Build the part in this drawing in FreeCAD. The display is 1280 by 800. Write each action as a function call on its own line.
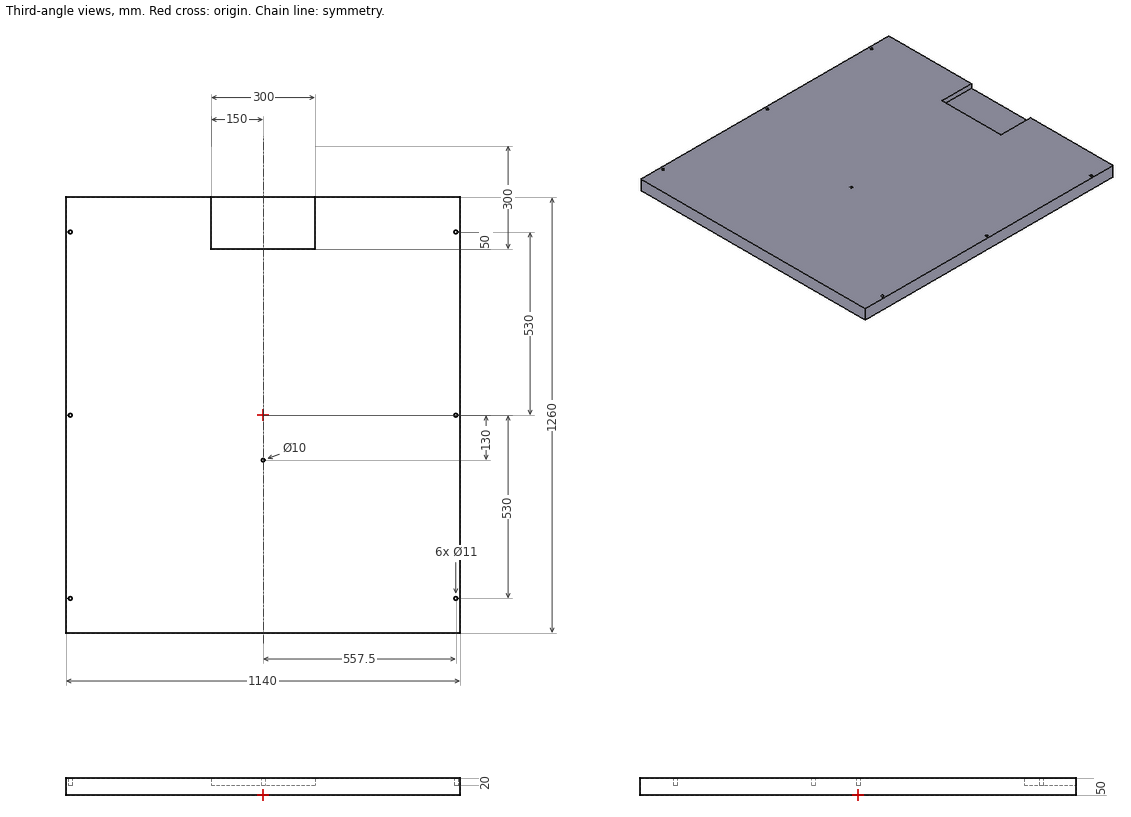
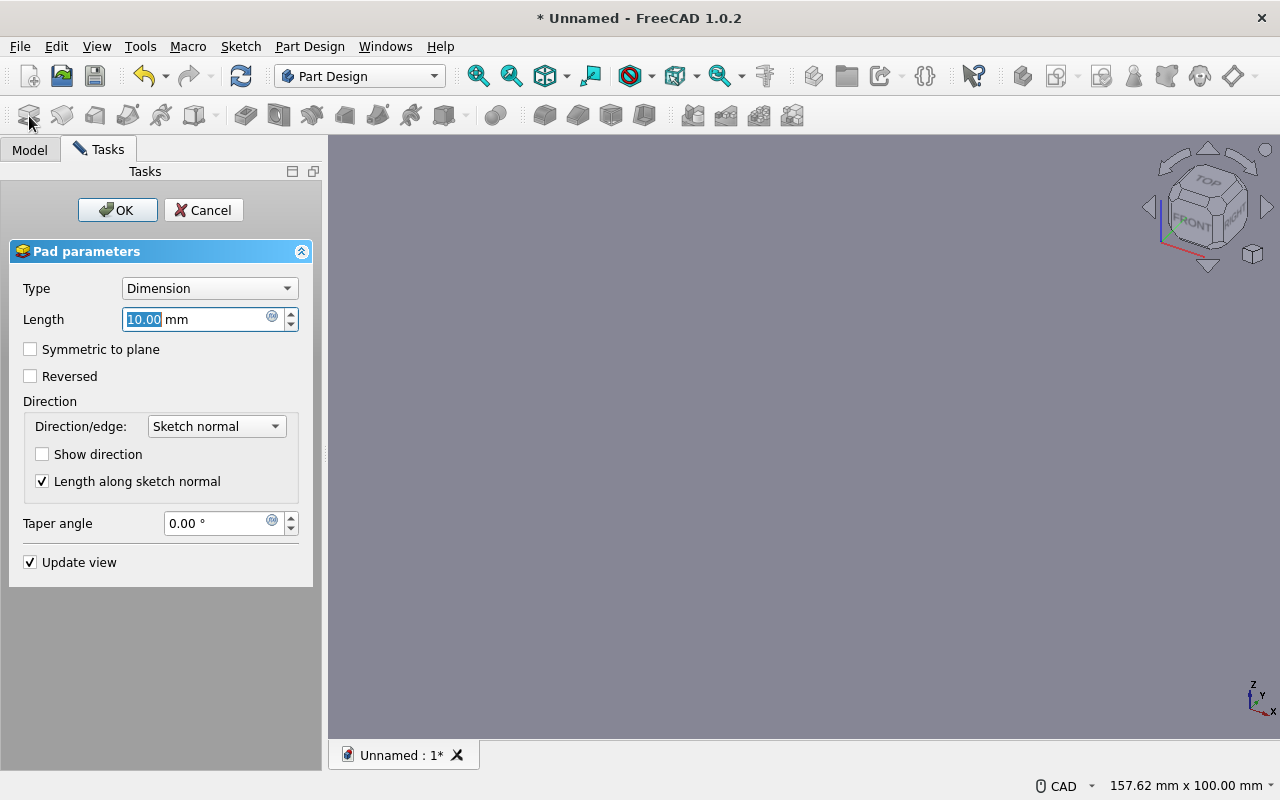
text(50)
key(Tab)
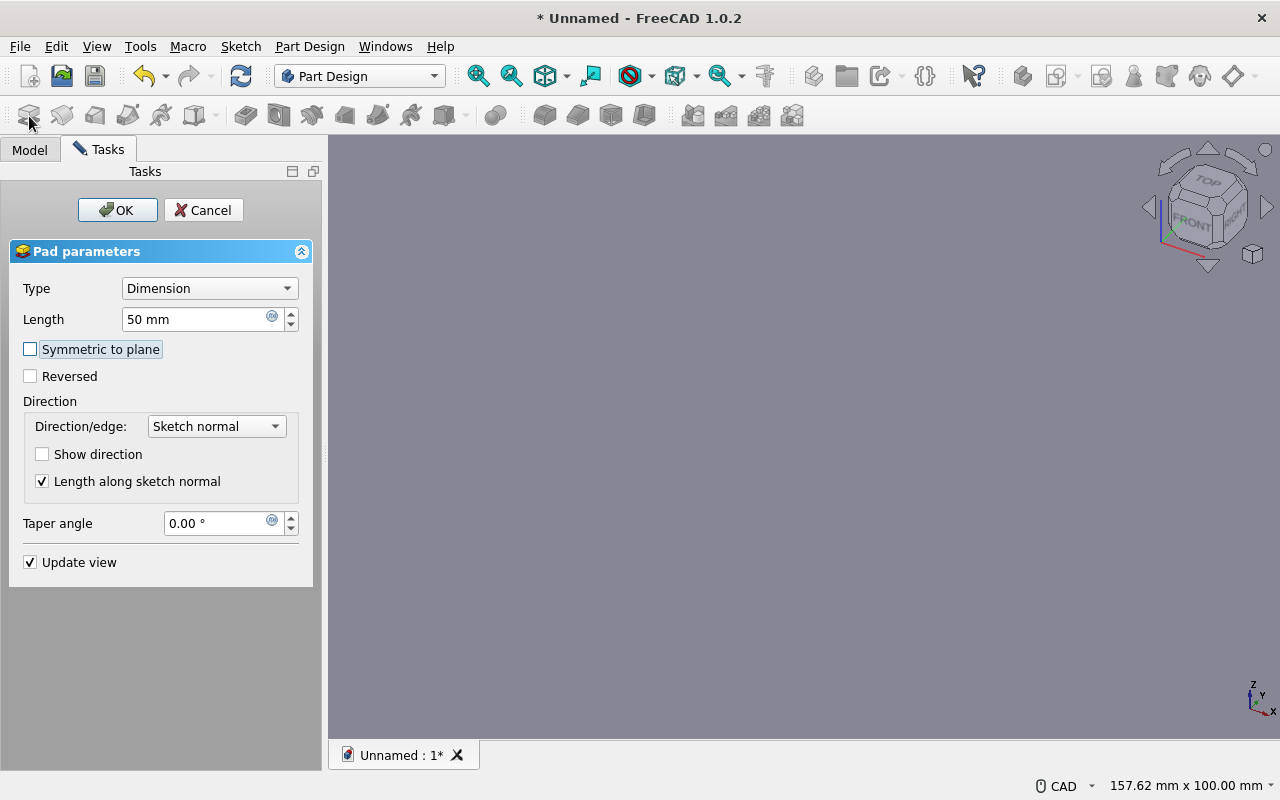
click(118, 210)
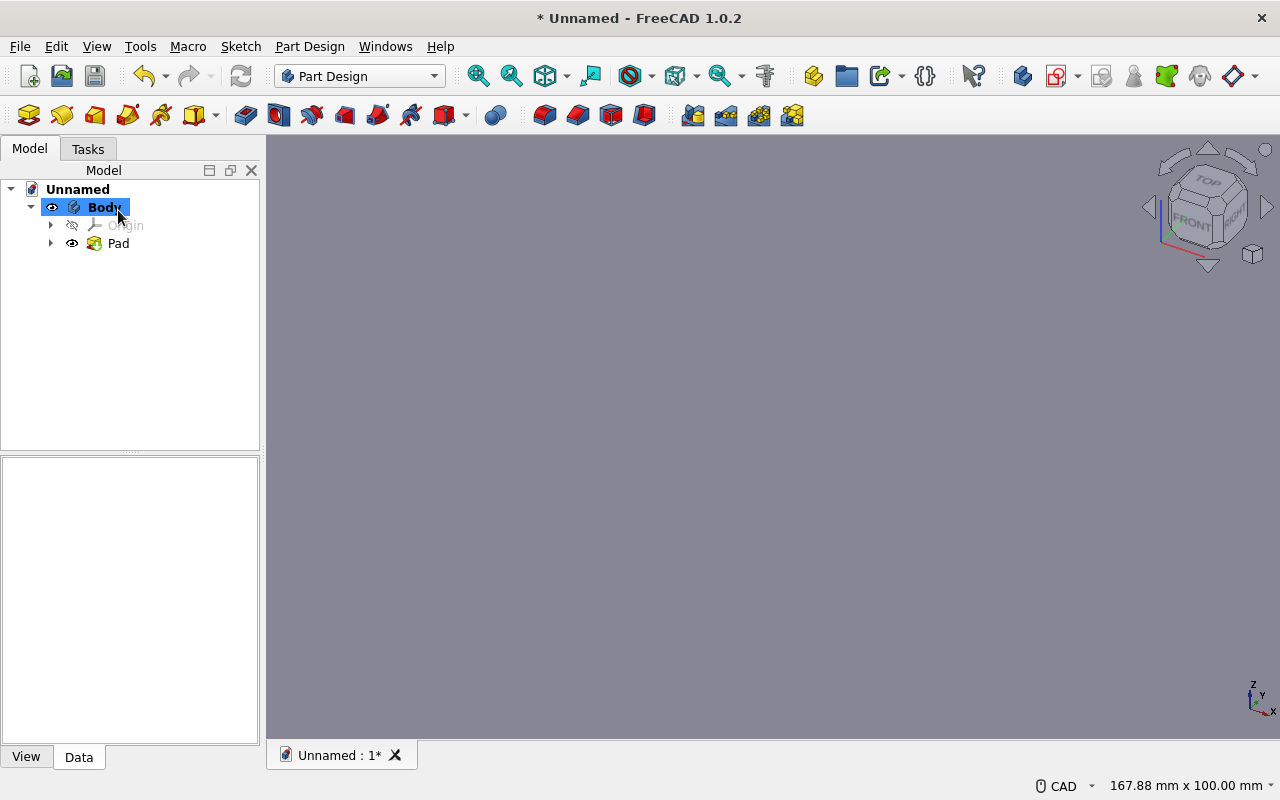
click(479, 76)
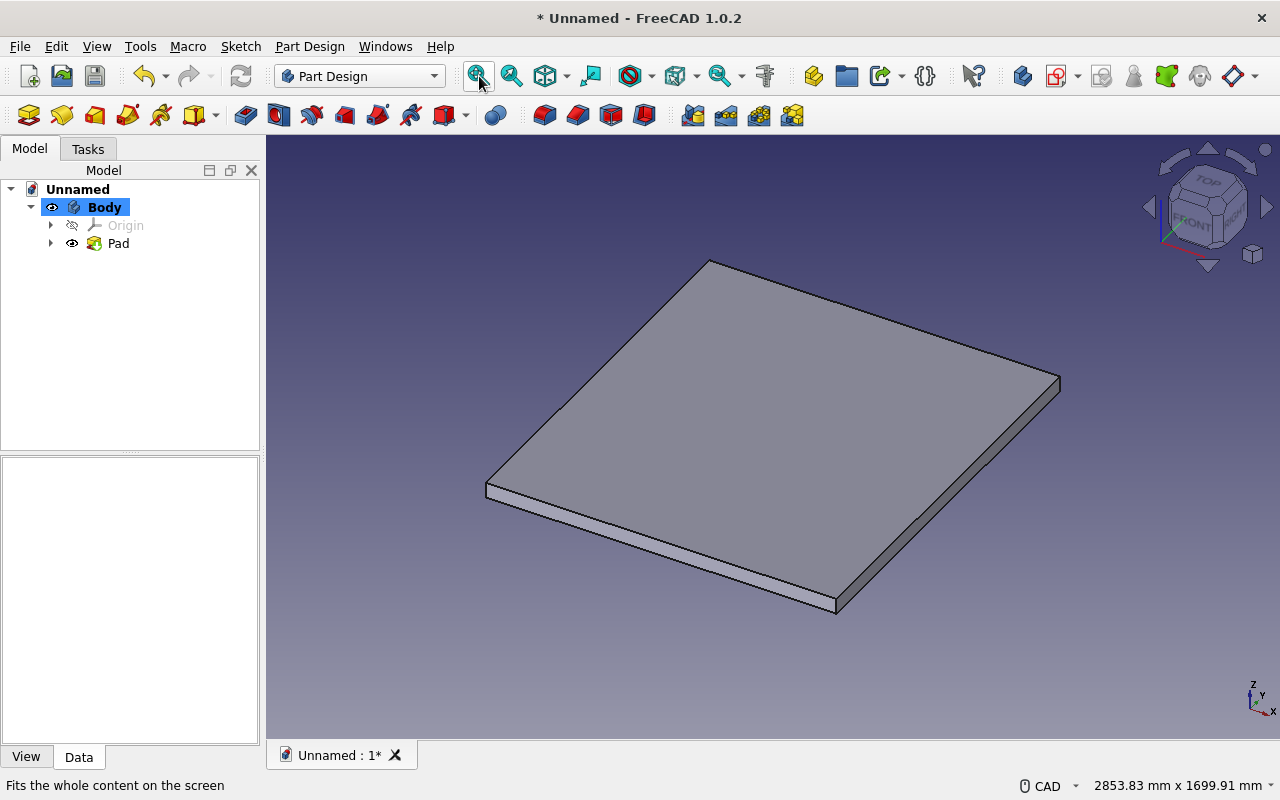
click(773, 429)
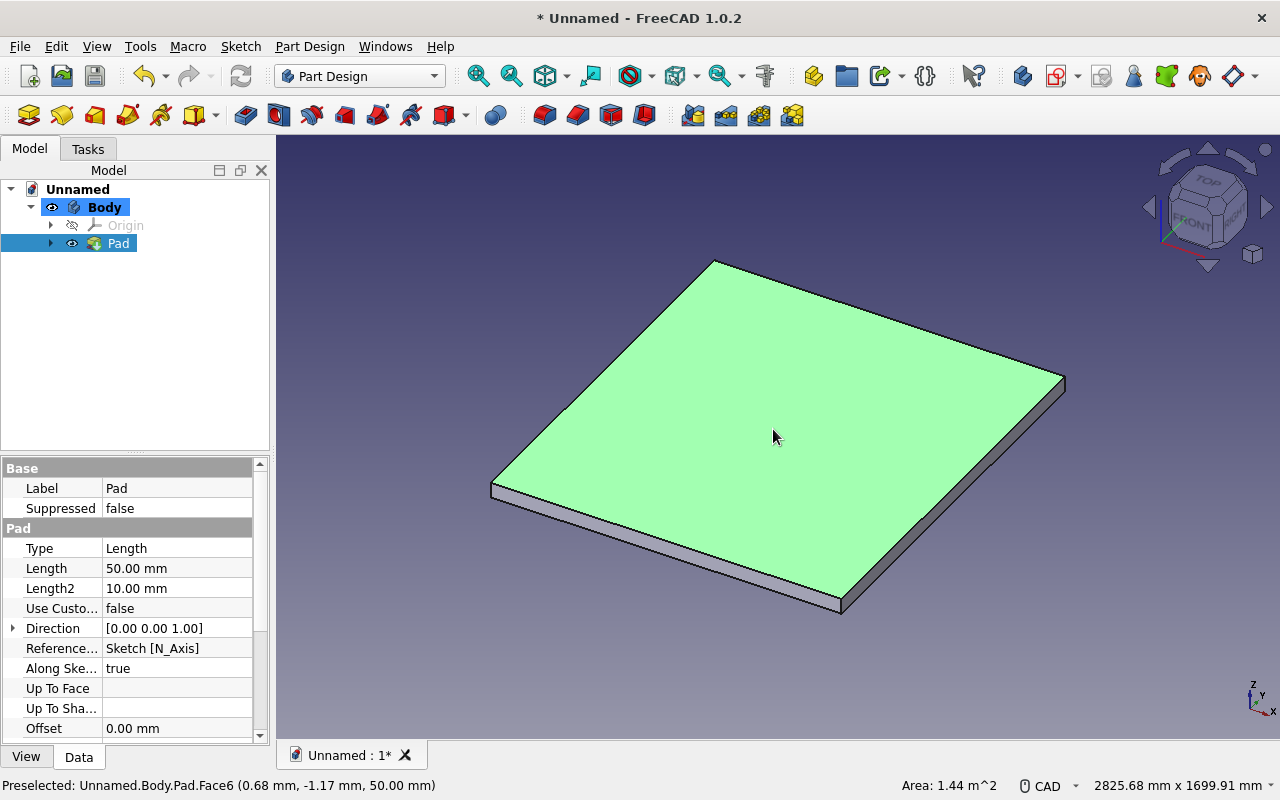
click(1056, 76)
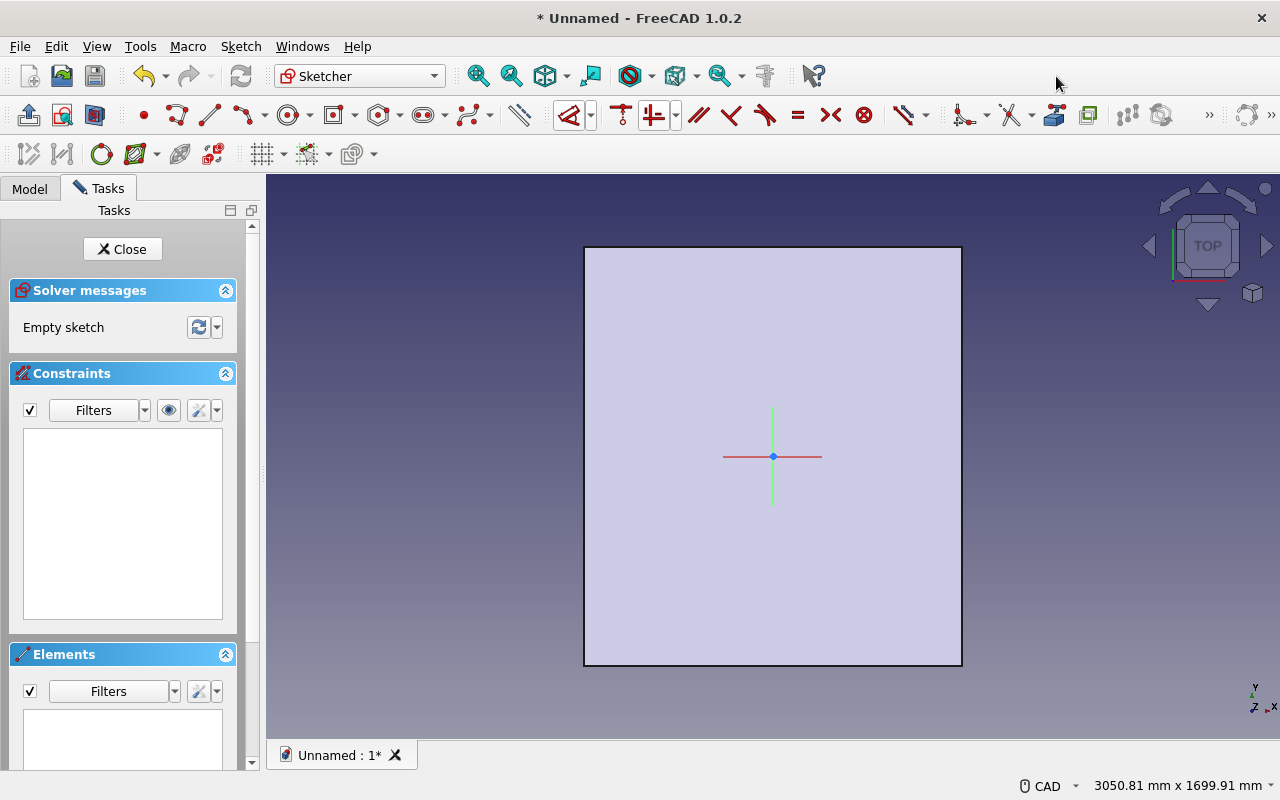
scroll(395, 640, down, 1)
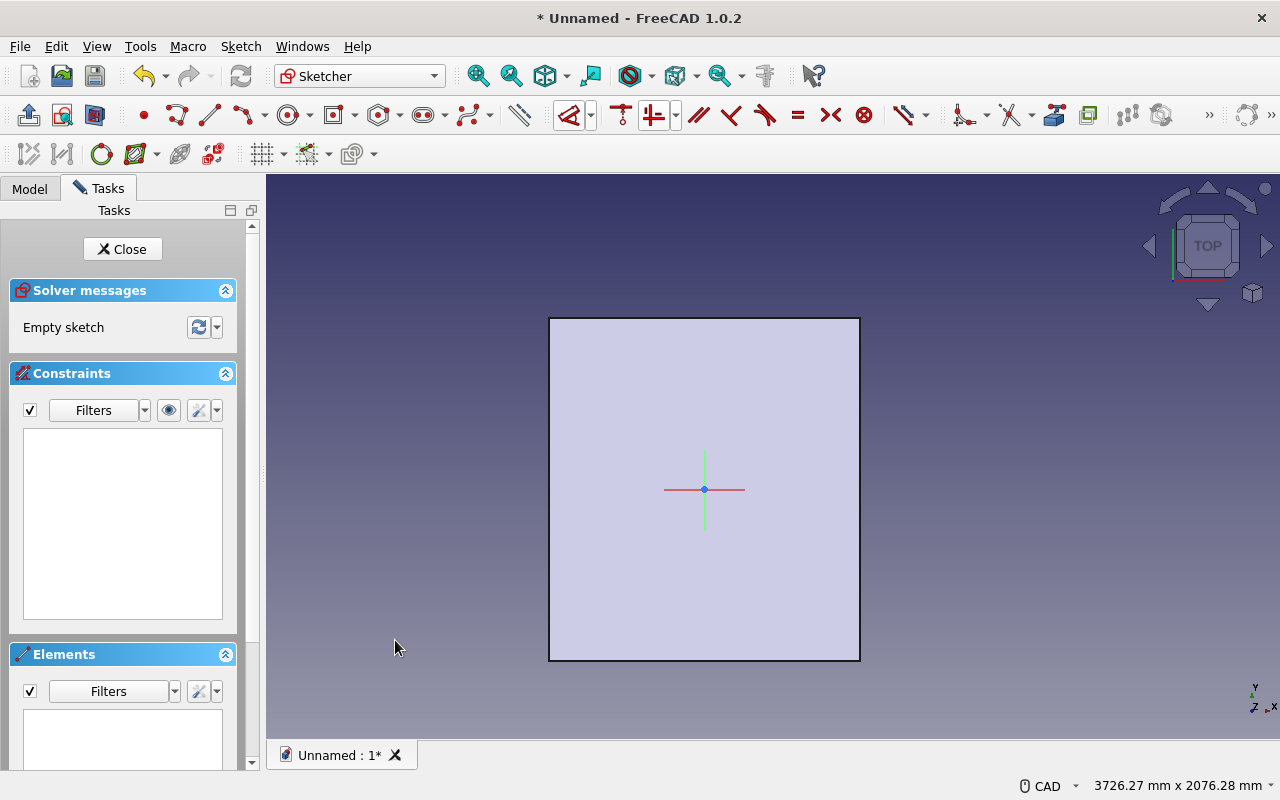
key(g)
key(r)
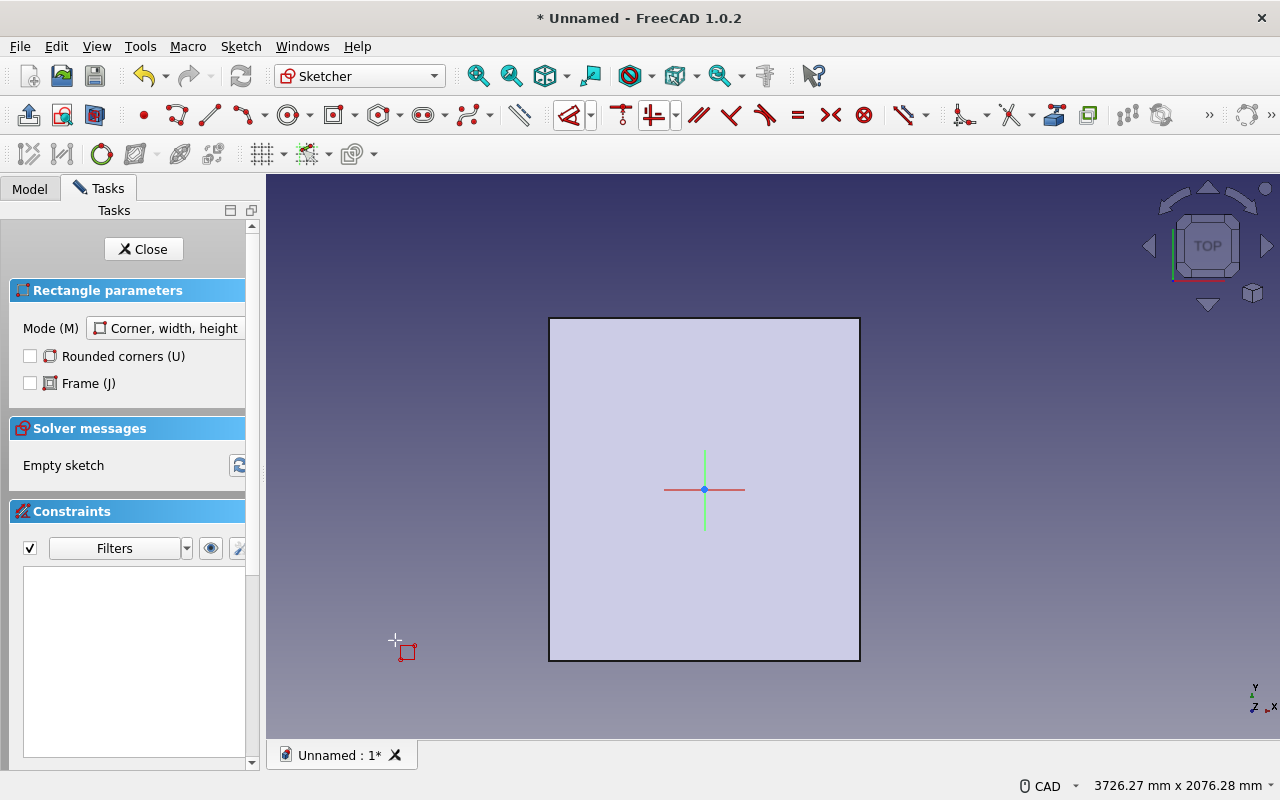
click(664, 278)
move(745, 359)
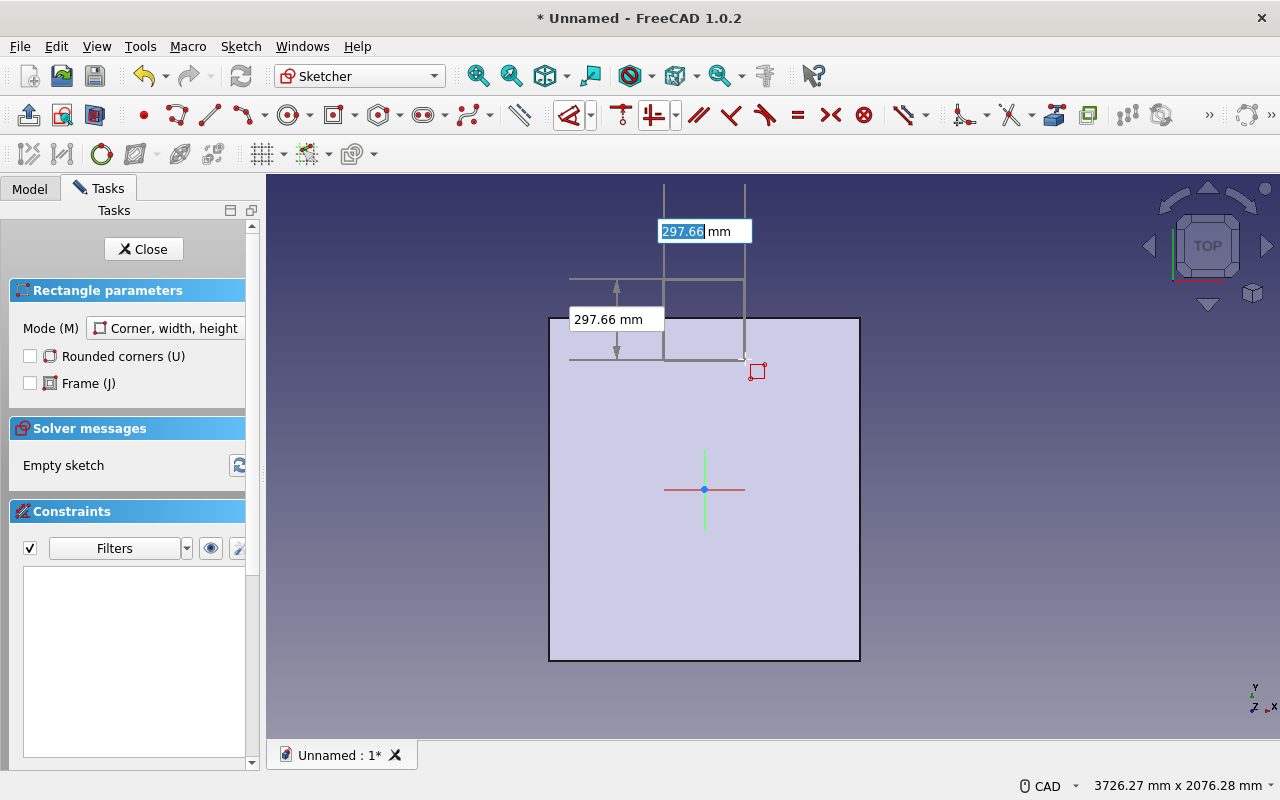
text(300)
key(Tab)
text(300)
key(Return)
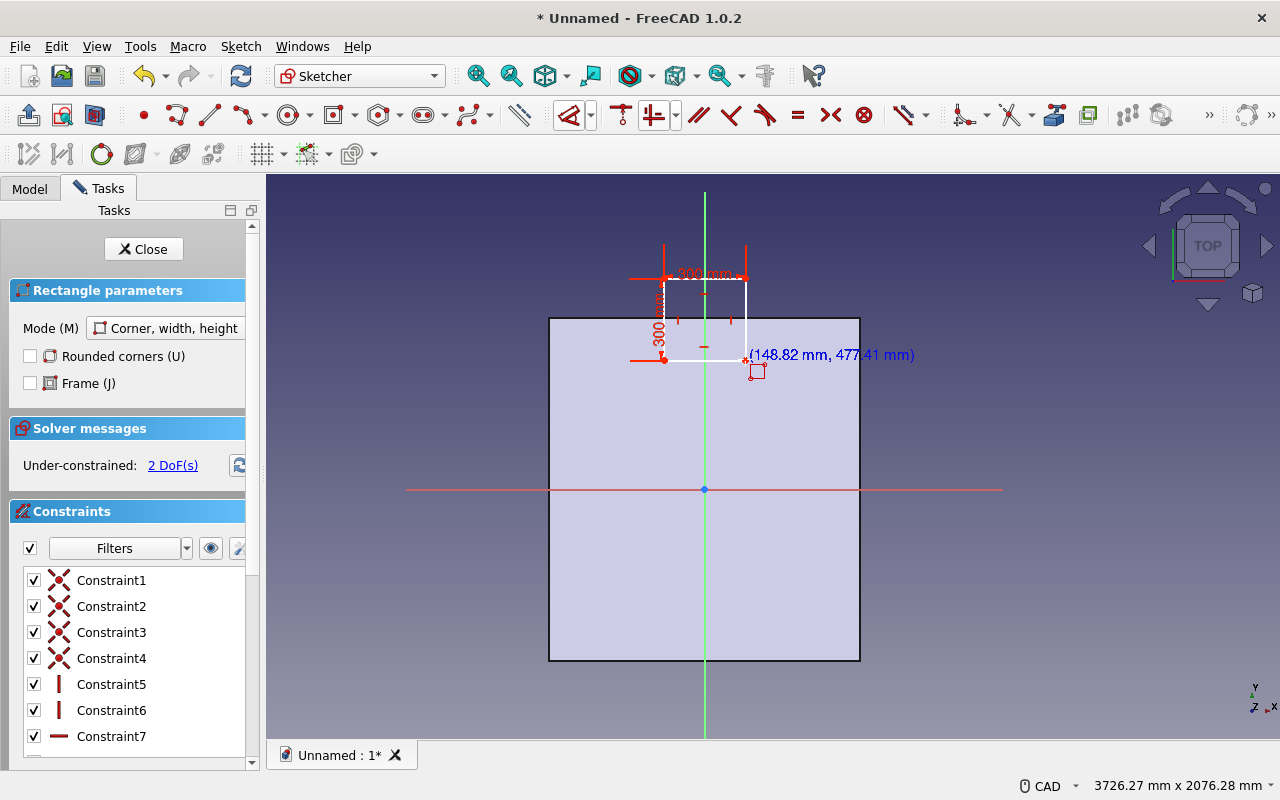
click(288, 116)